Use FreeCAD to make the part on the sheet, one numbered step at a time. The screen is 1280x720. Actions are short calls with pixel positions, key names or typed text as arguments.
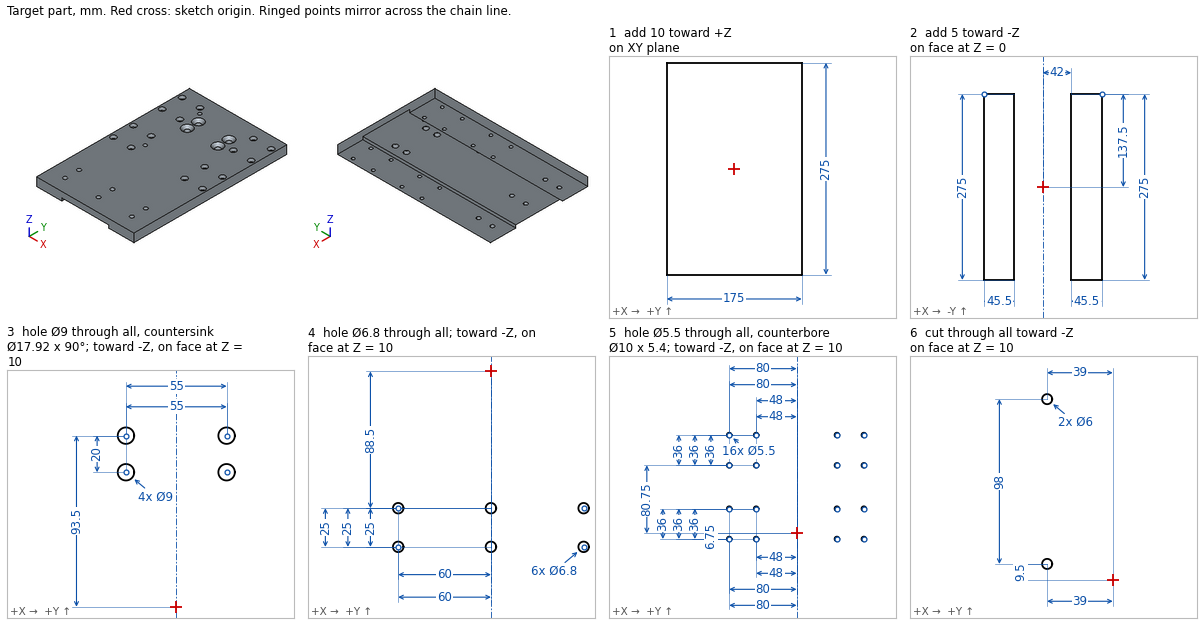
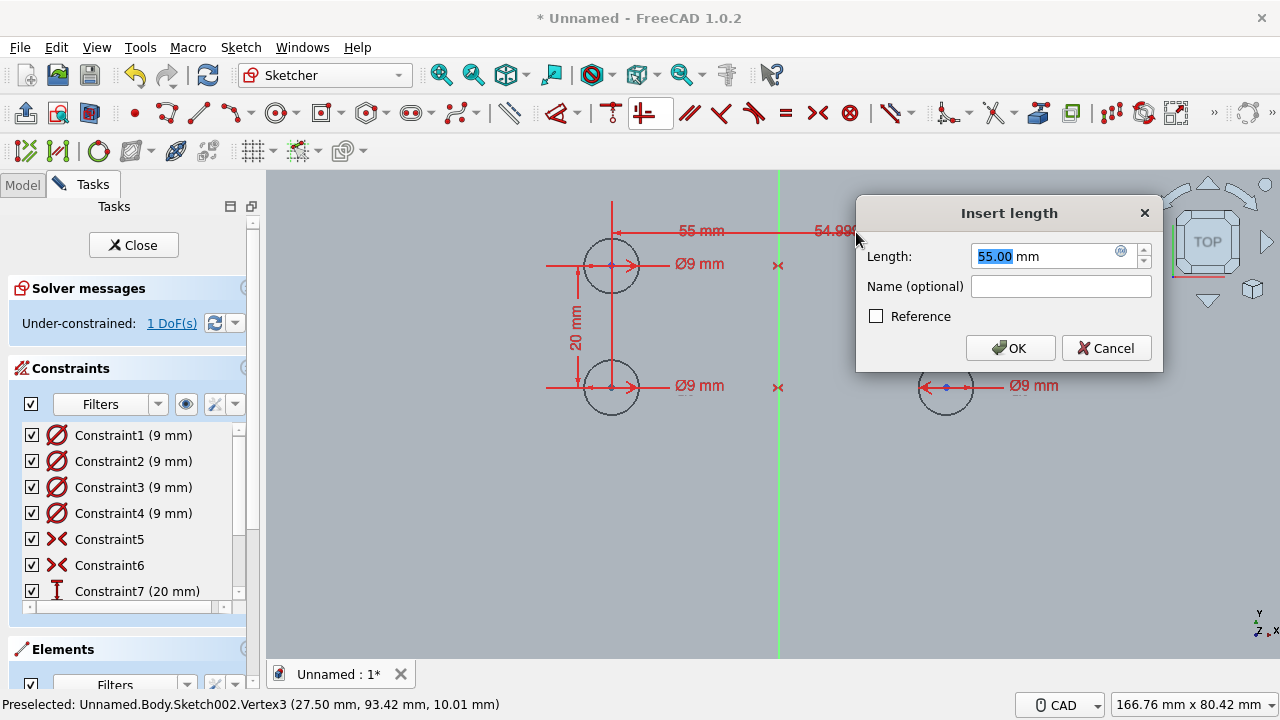
text(55)
key(Return)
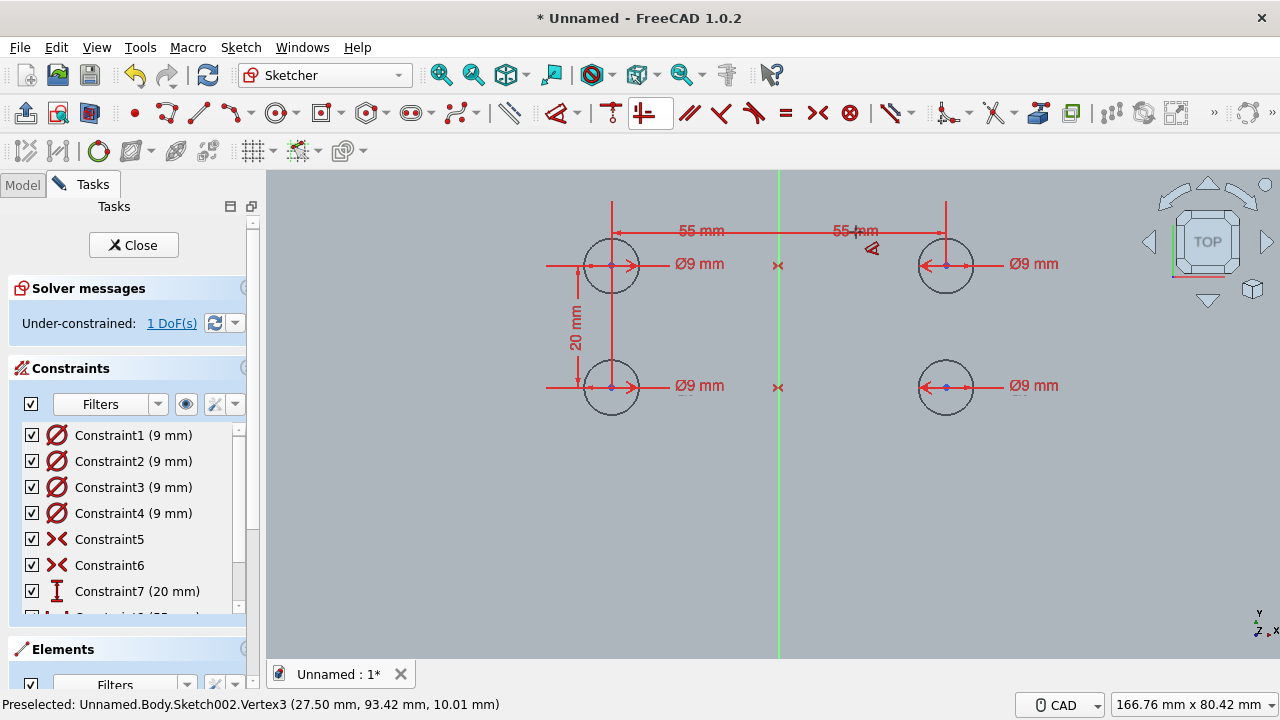
click(612, 266)
click(578, 448)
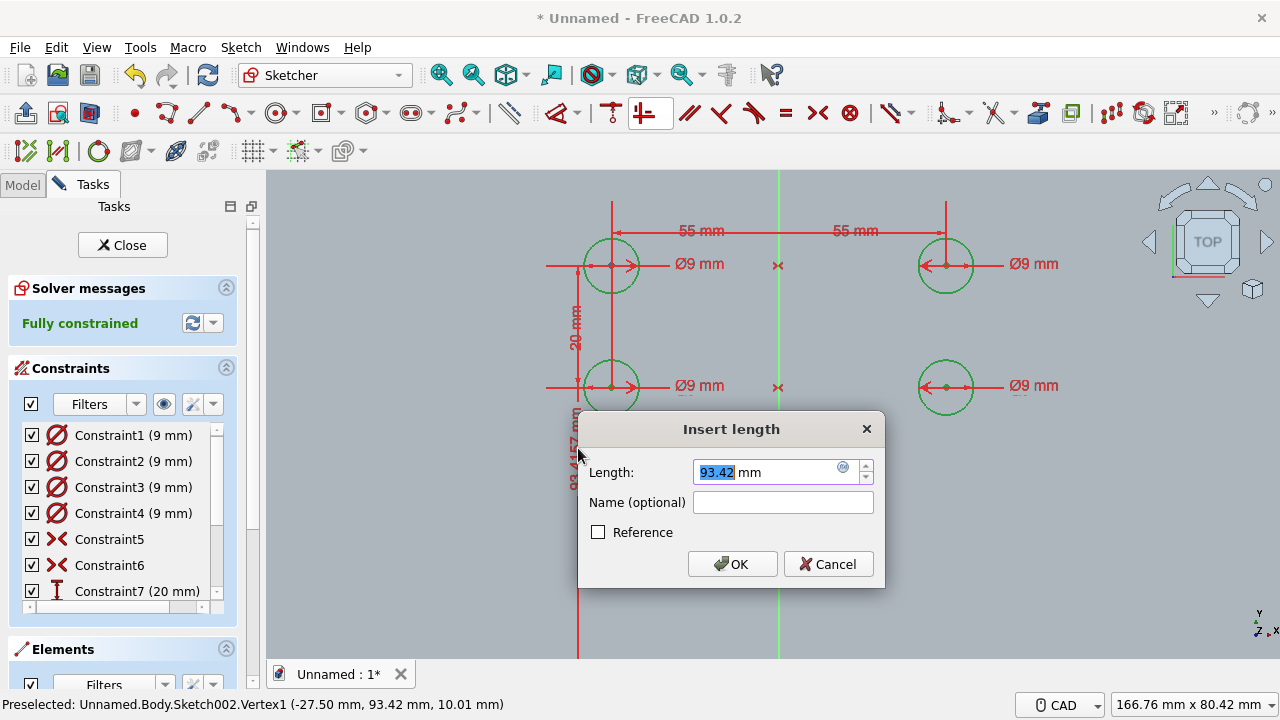
text(93.5)
key(Return)
key(Escape)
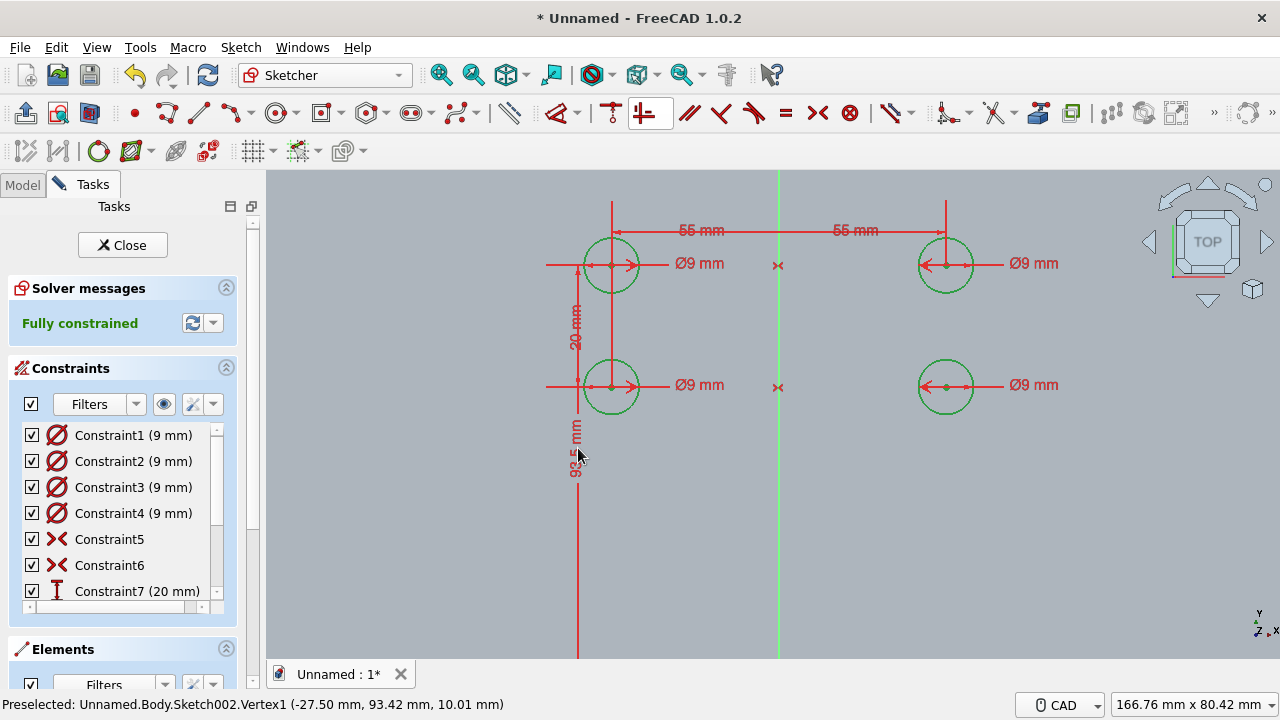
click(123, 245)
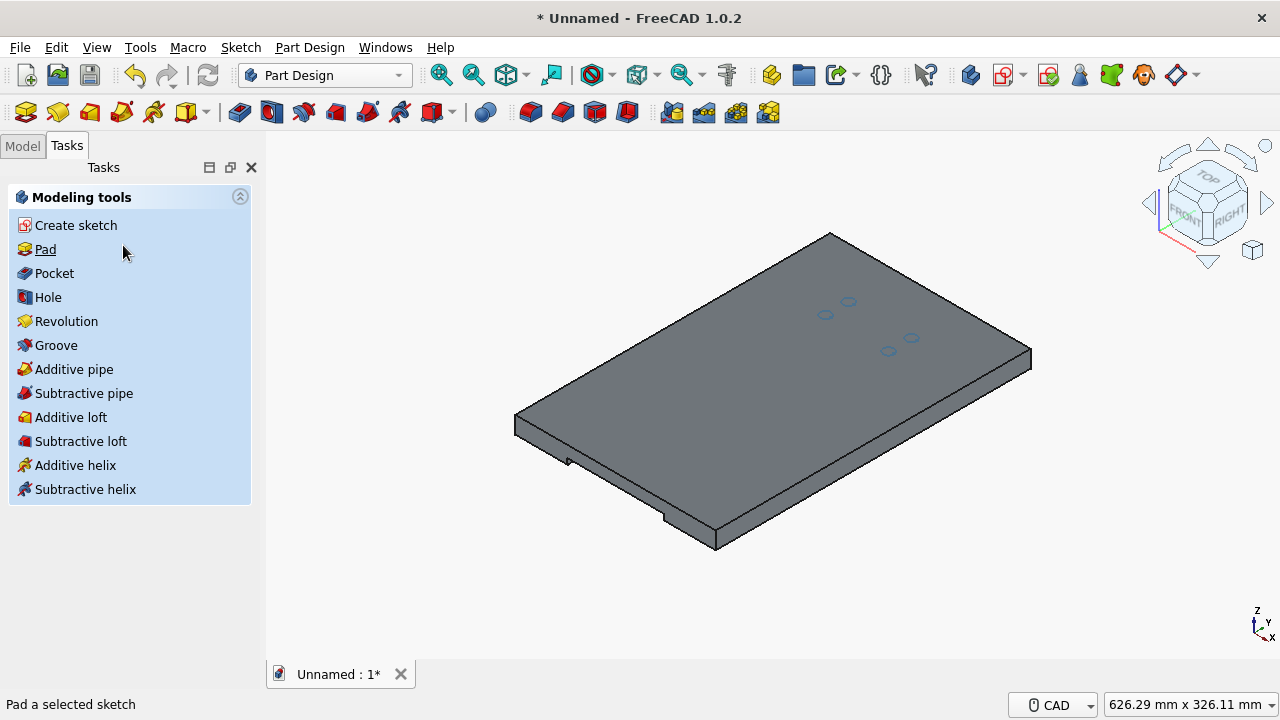
click(272, 112)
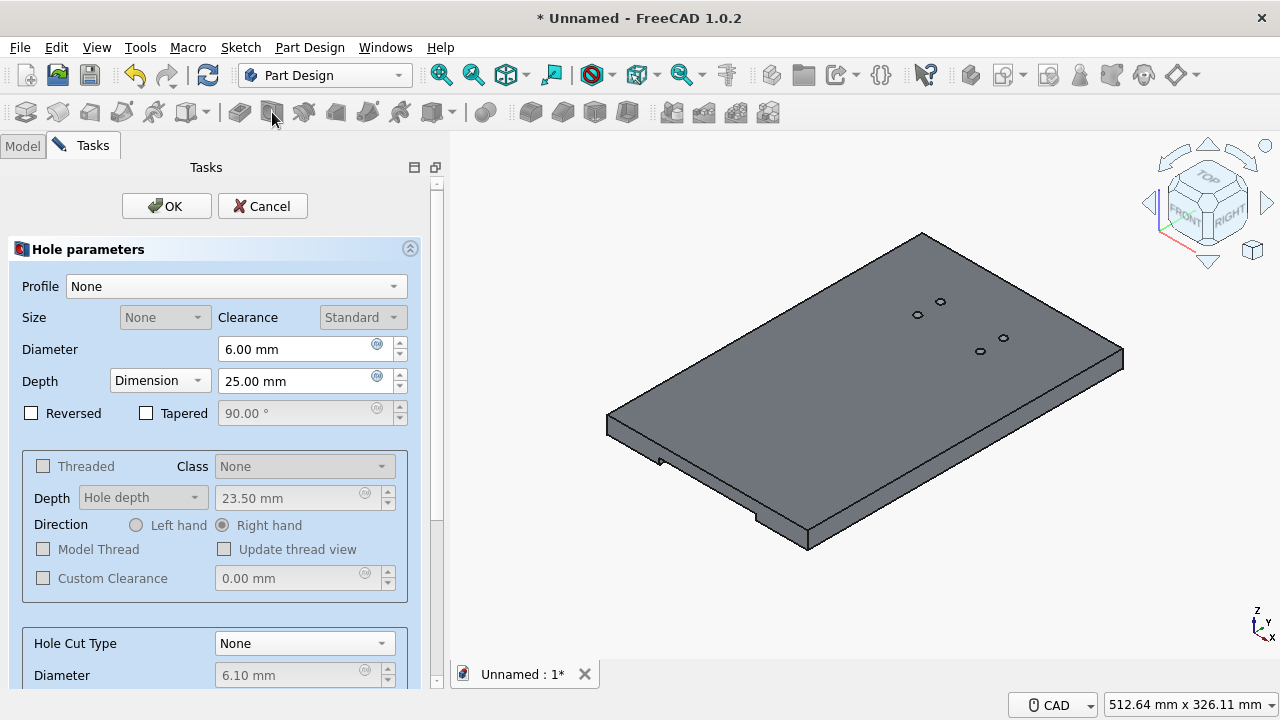
triple_click(305, 349)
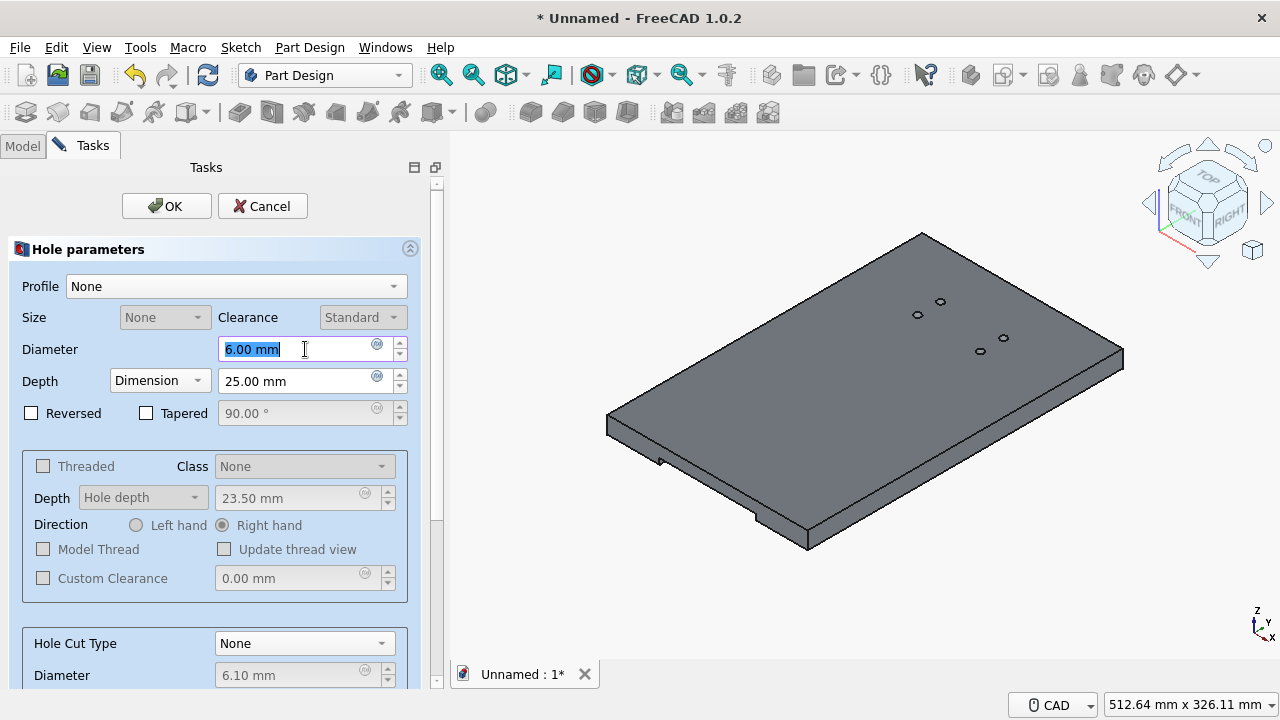
text(9)
key(Tab)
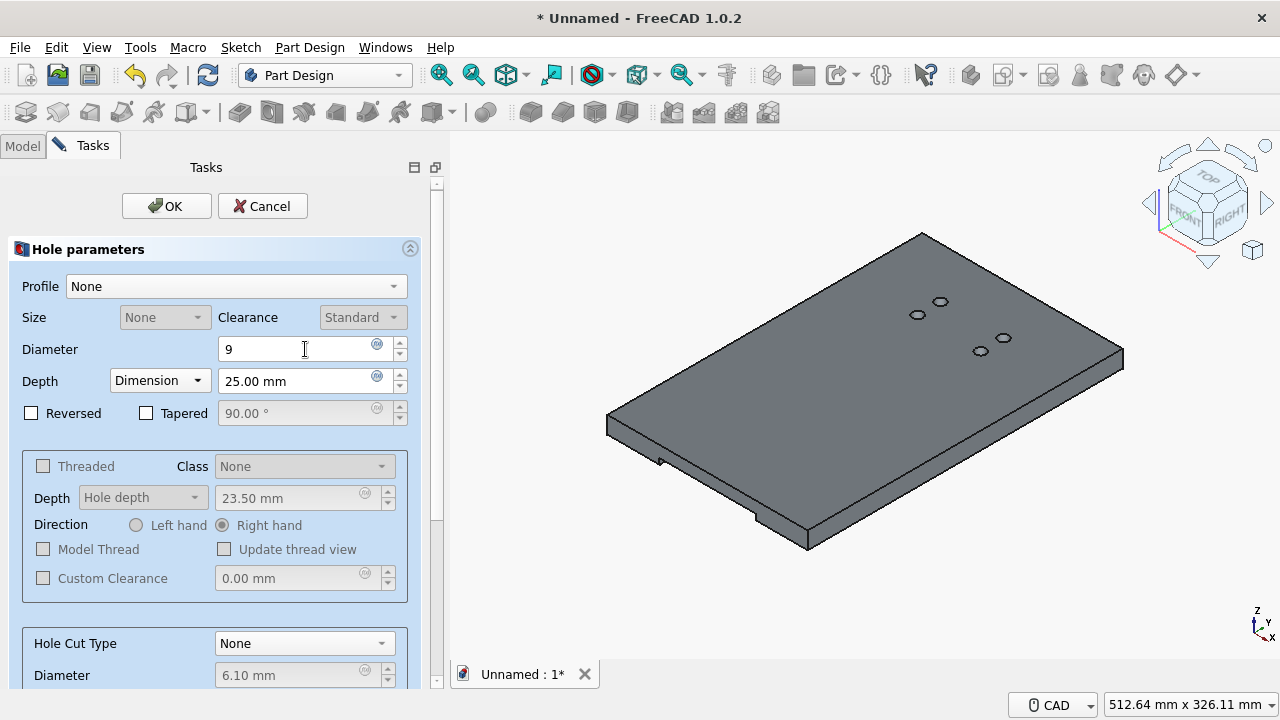
click(161, 380)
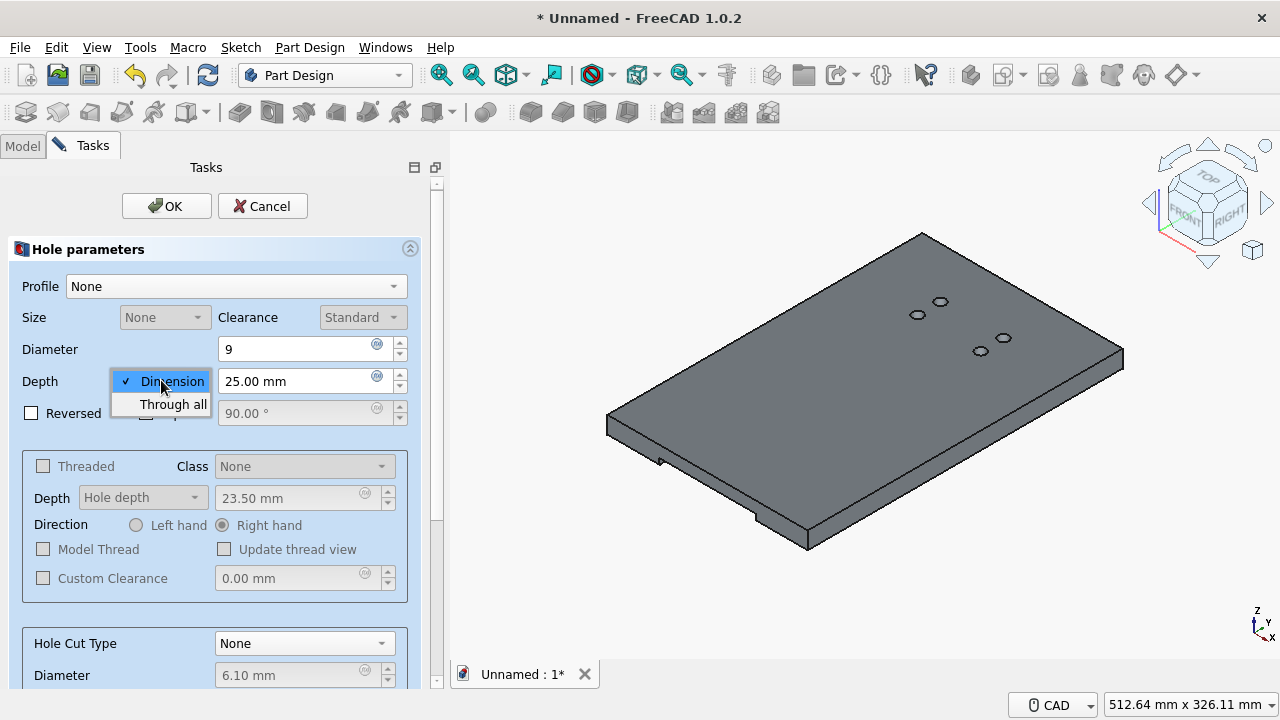
click(160, 404)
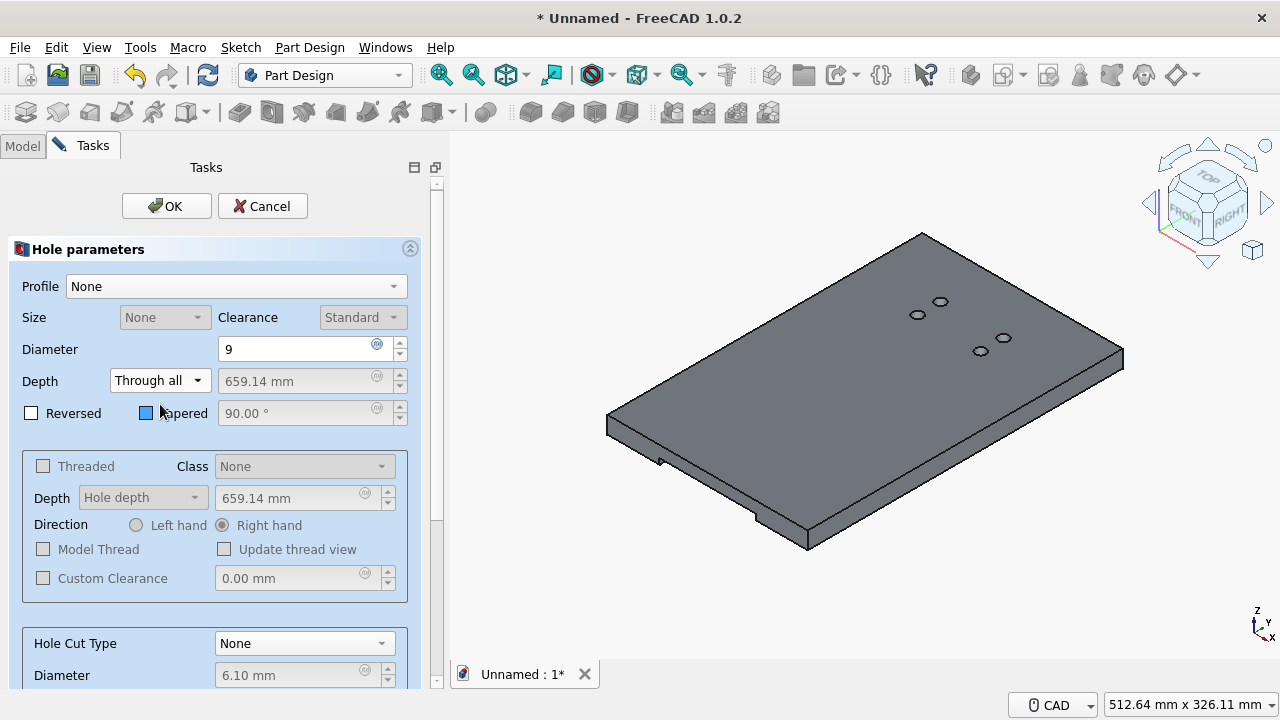
click(306, 644)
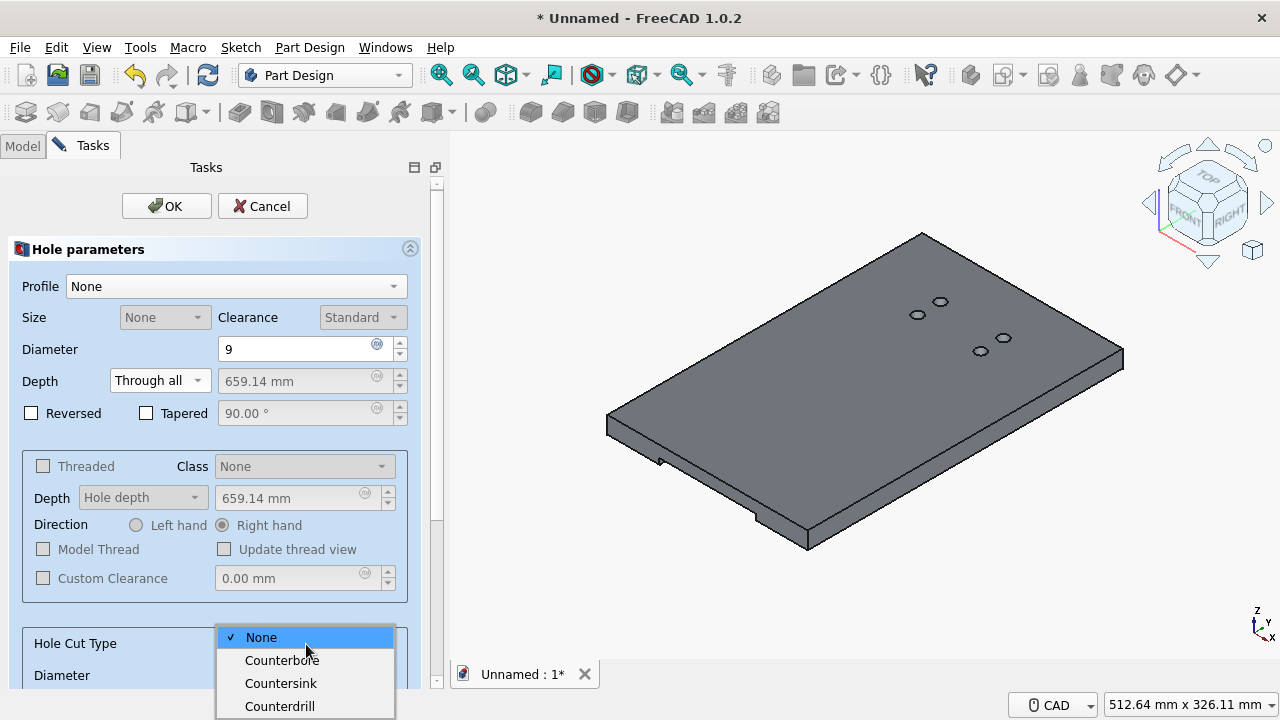
click(304, 684)